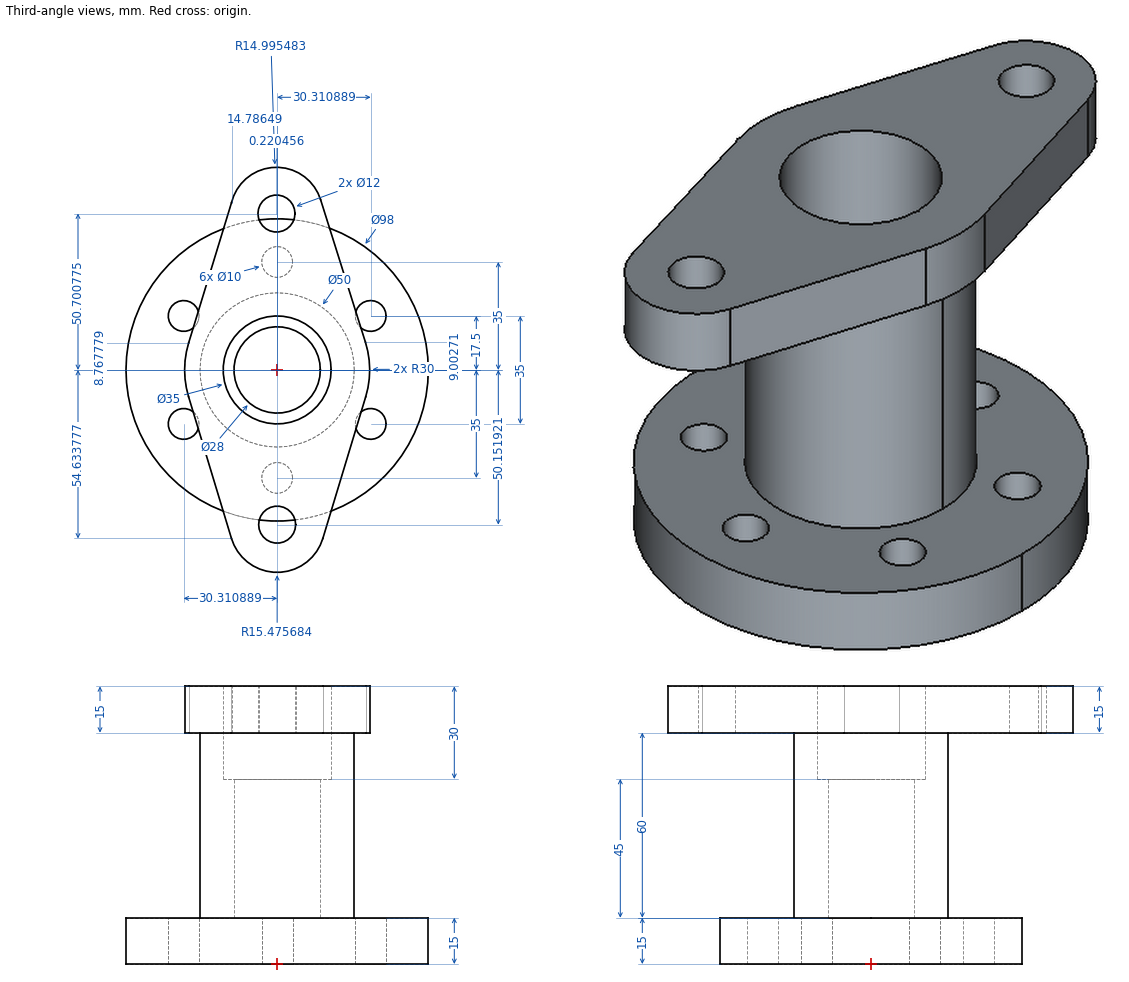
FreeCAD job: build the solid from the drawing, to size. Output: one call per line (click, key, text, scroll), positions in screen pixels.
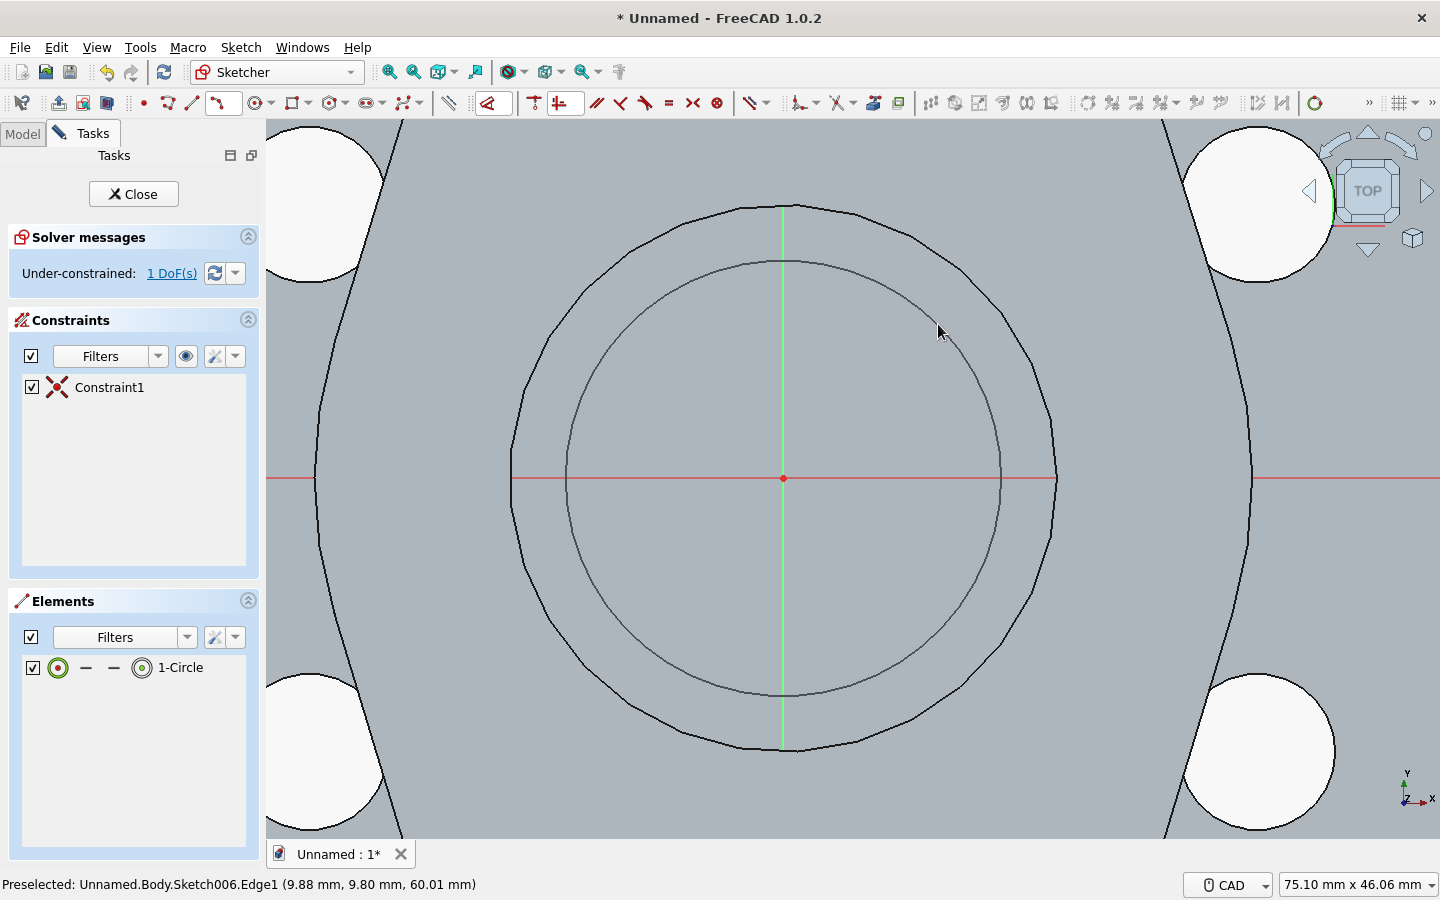
click(937, 324)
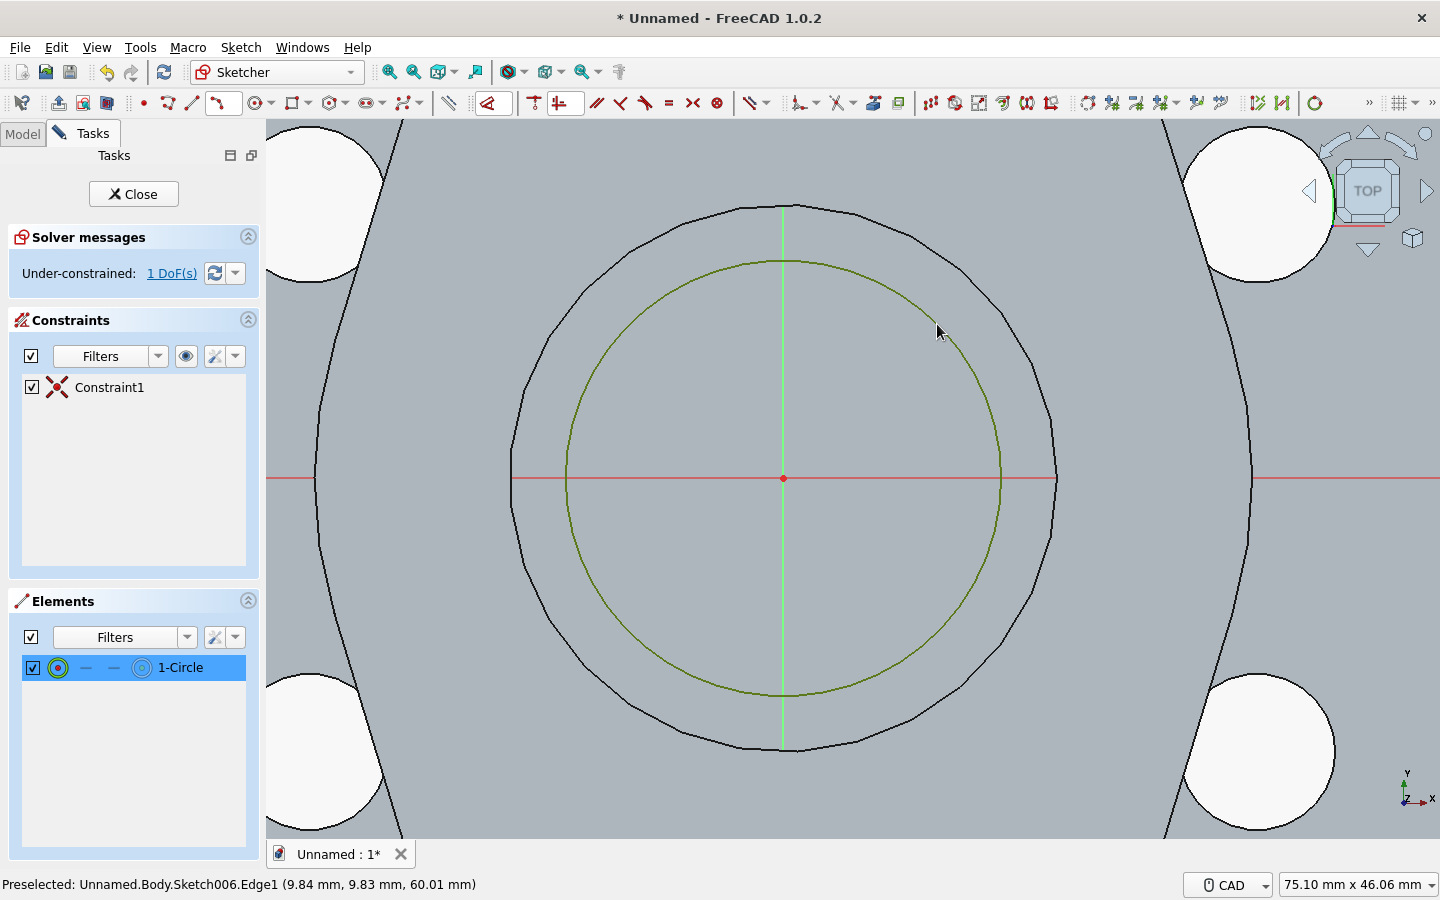
click(506, 104)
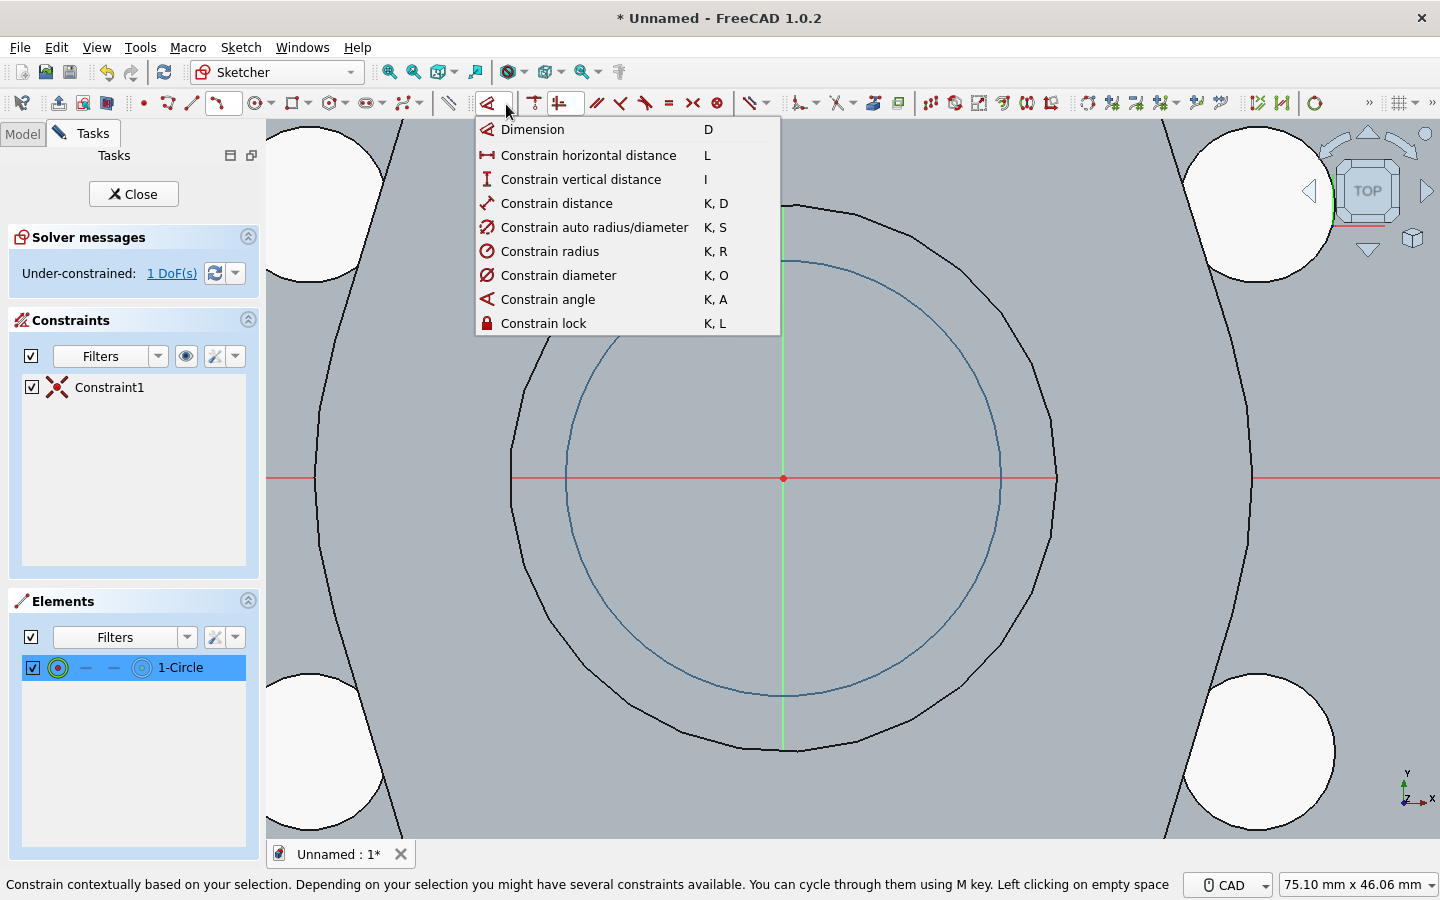
click(628, 275)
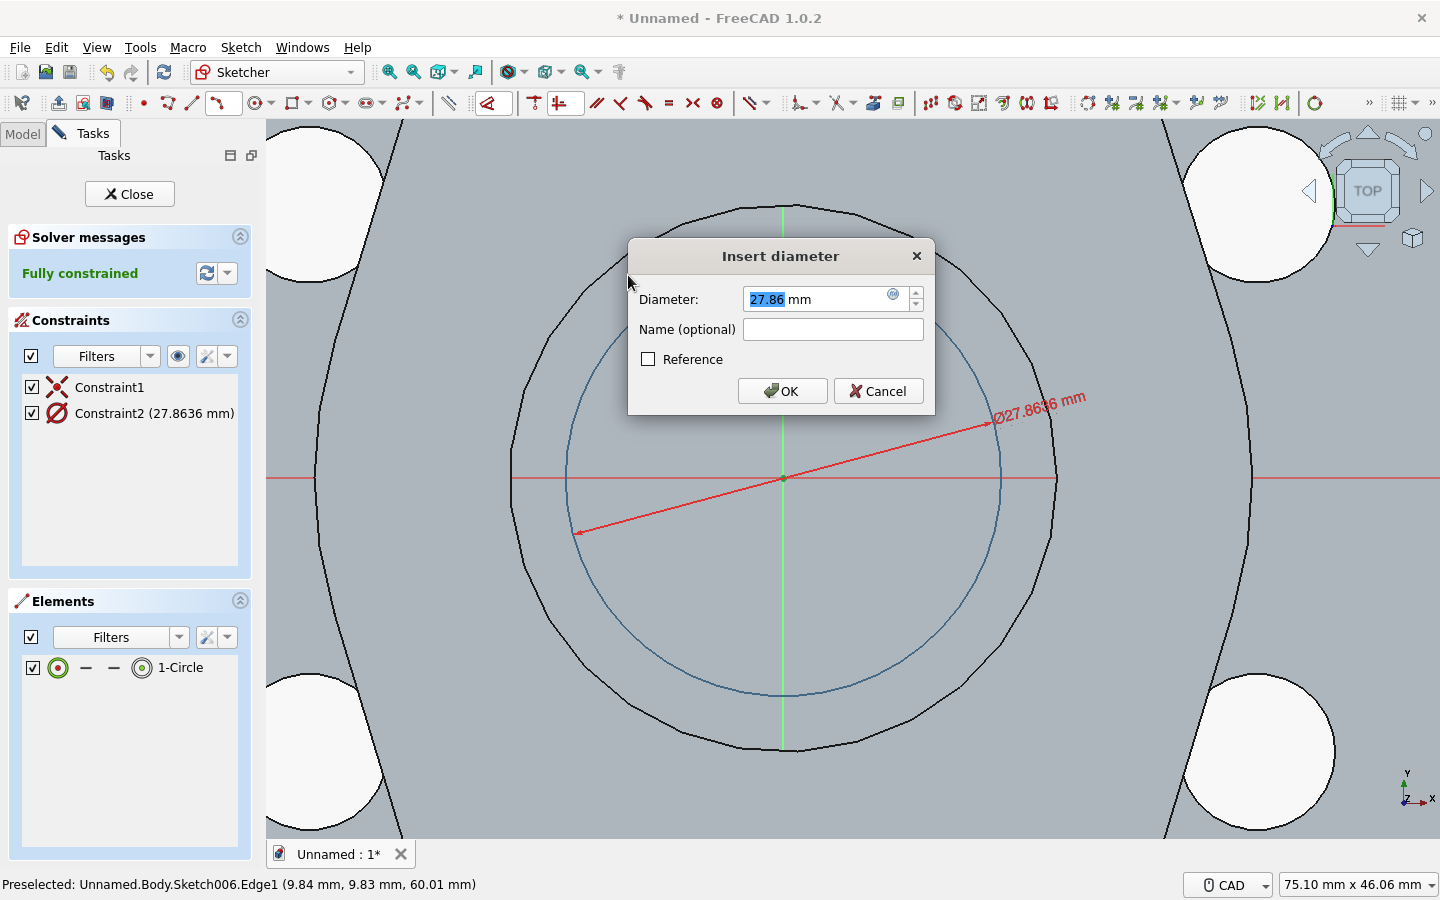
text(28)
key(Return)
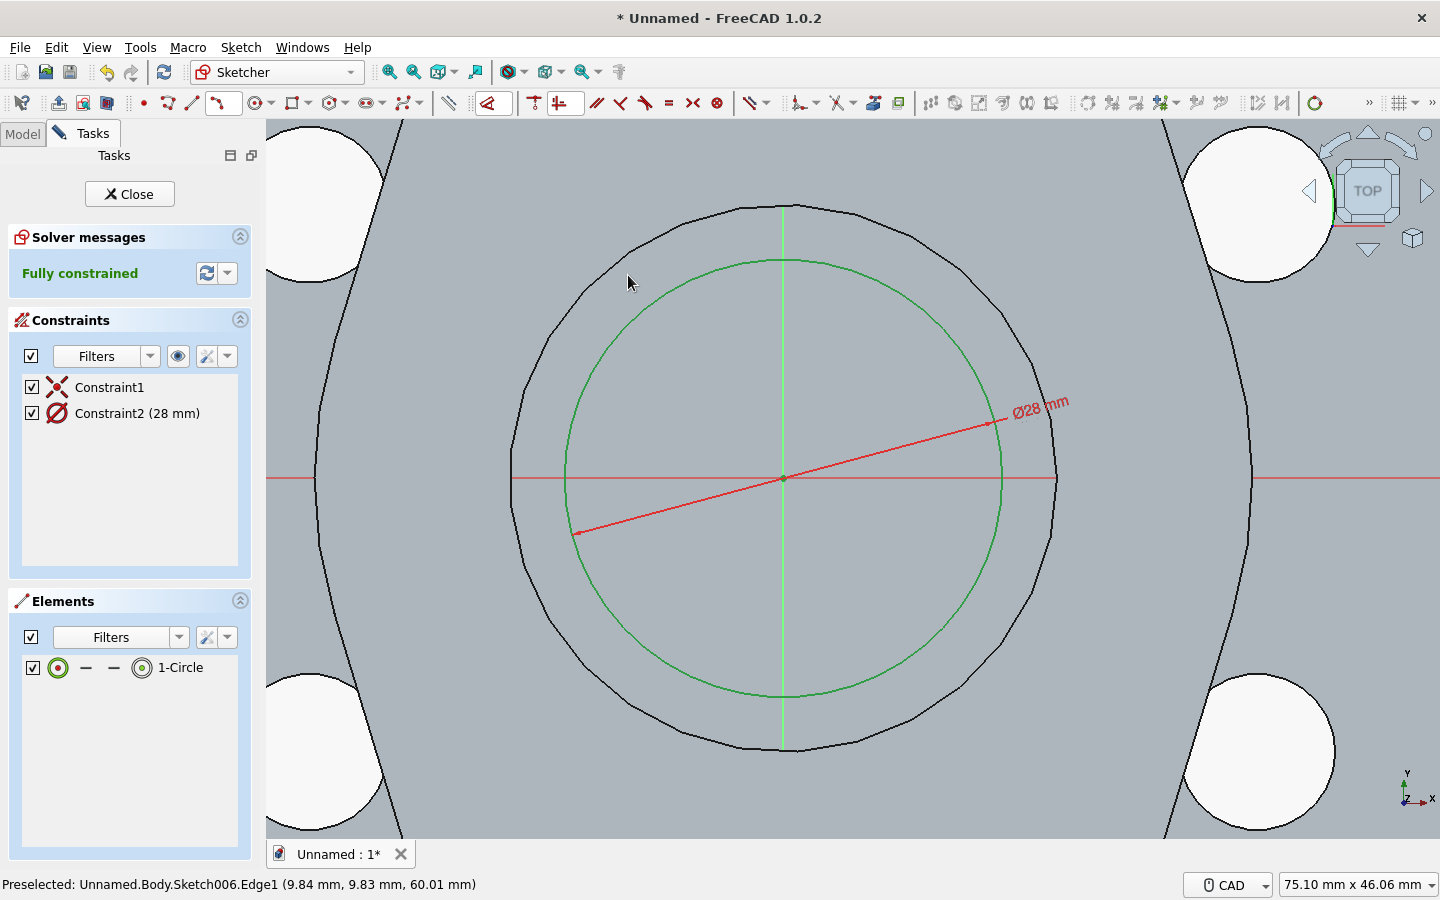
click(130, 194)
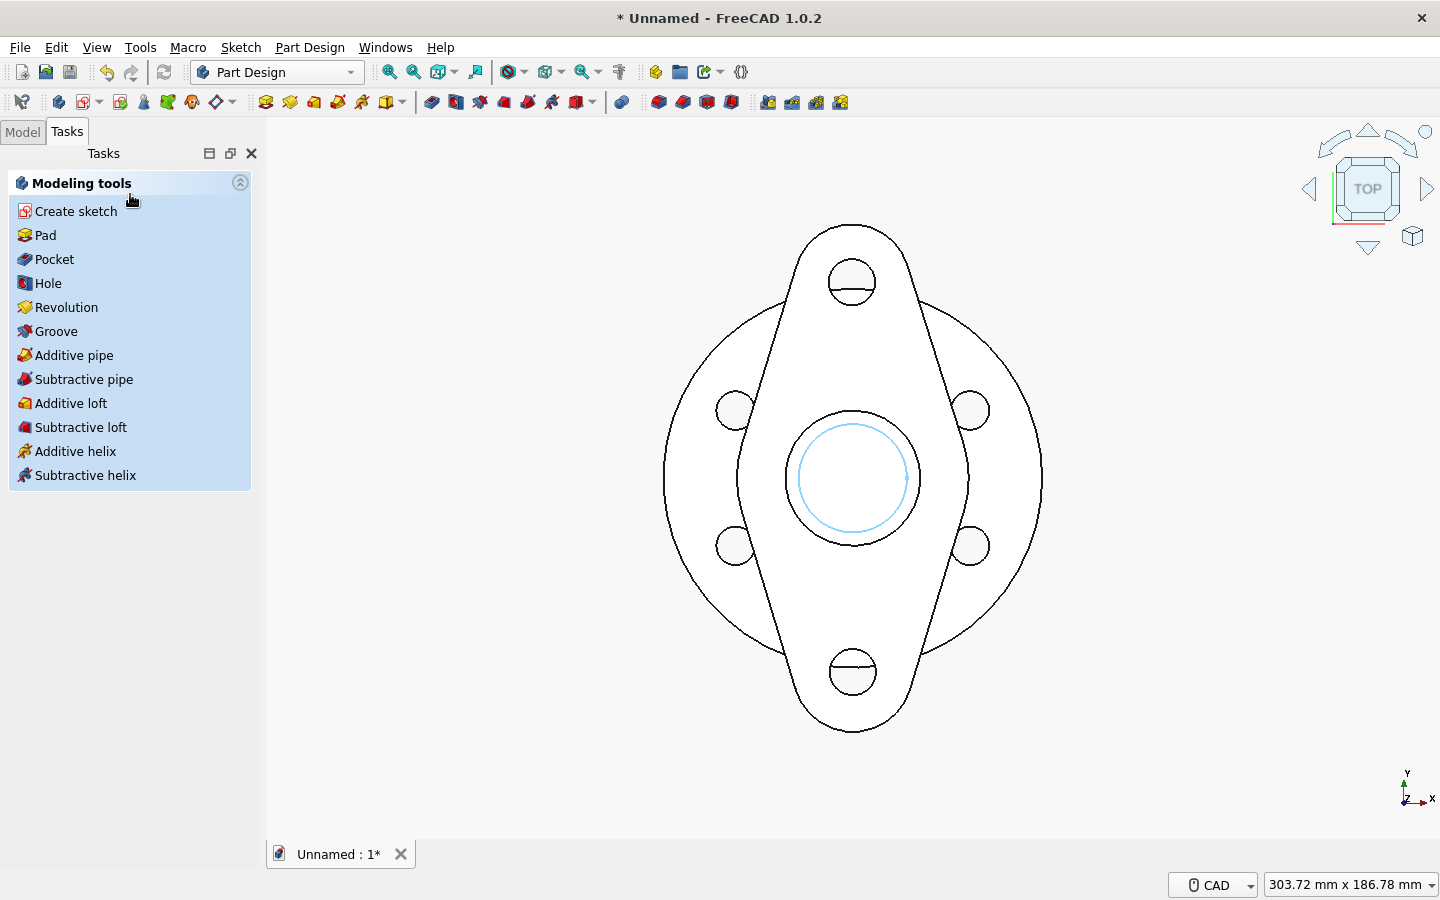
click(432, 102)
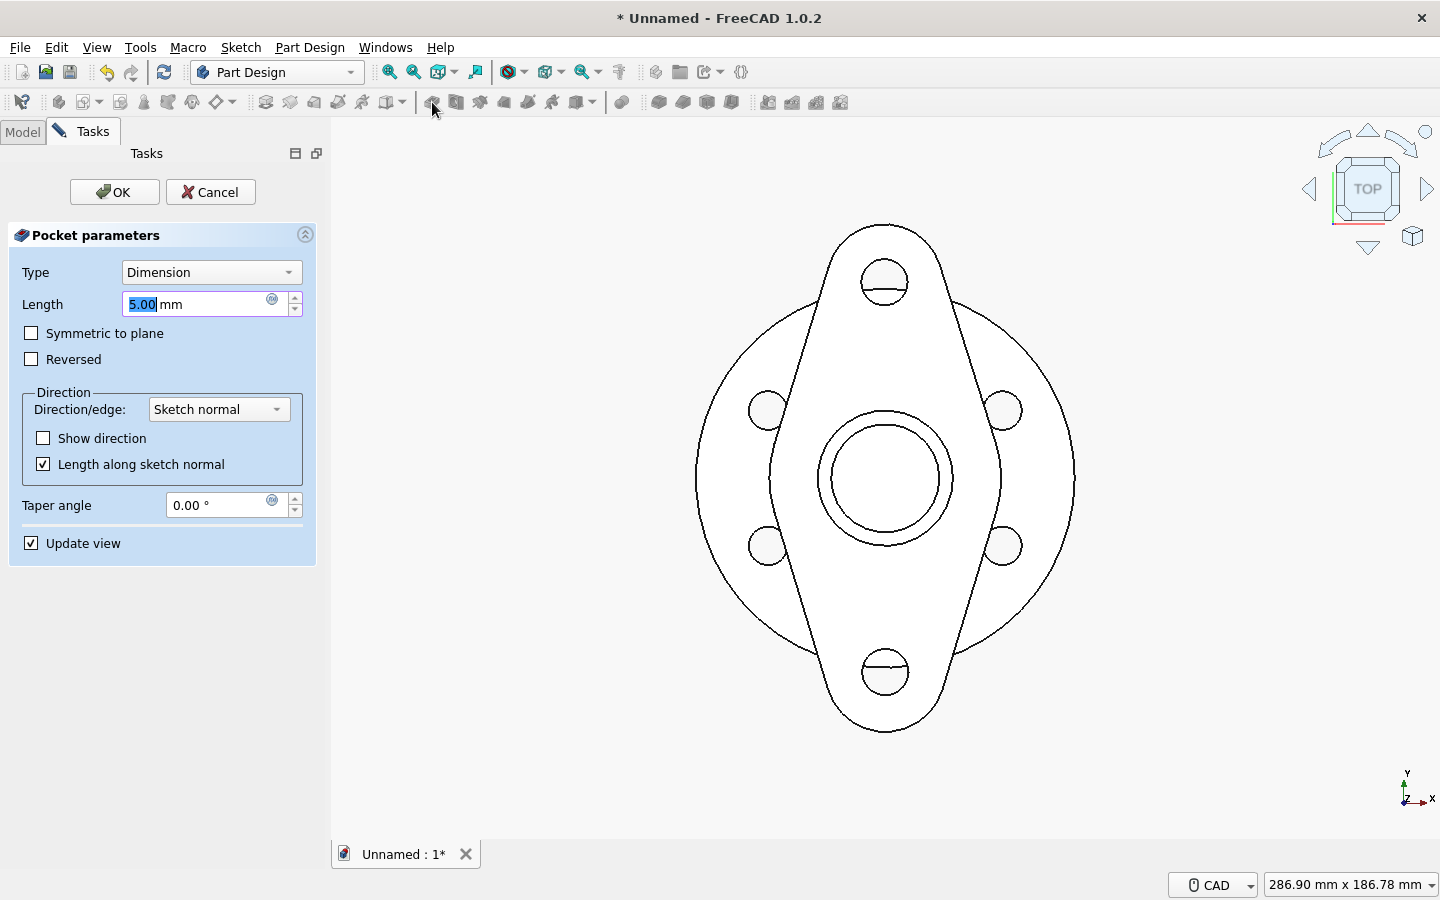
text(45)
key(Tab)